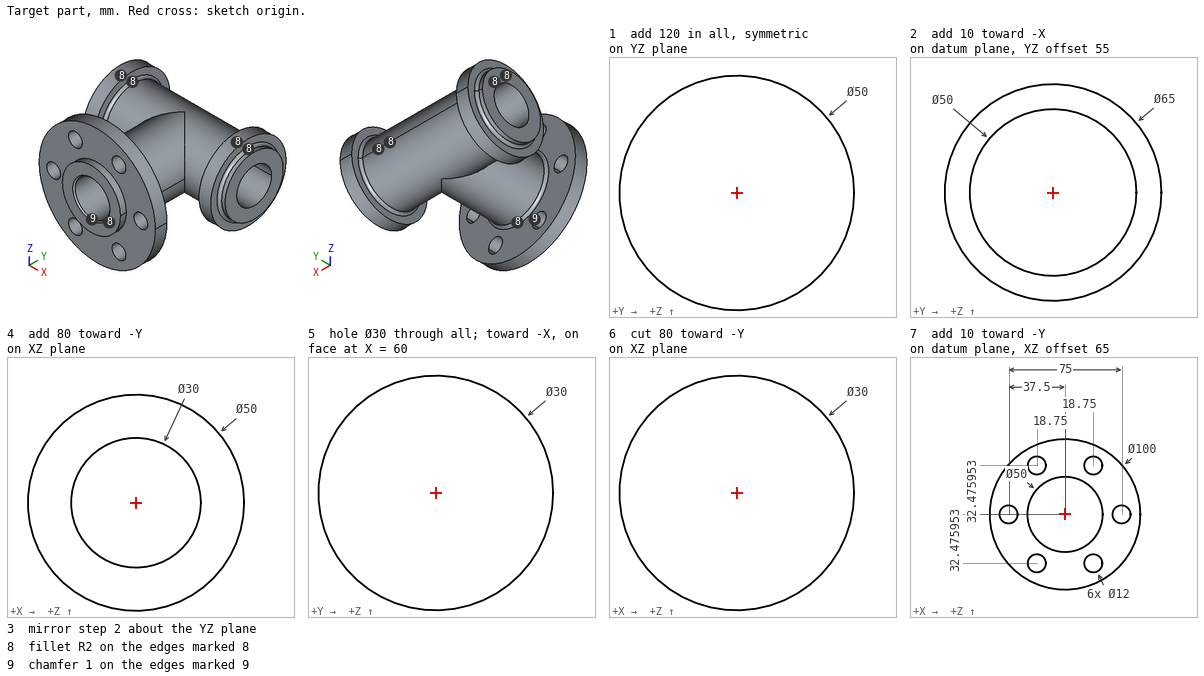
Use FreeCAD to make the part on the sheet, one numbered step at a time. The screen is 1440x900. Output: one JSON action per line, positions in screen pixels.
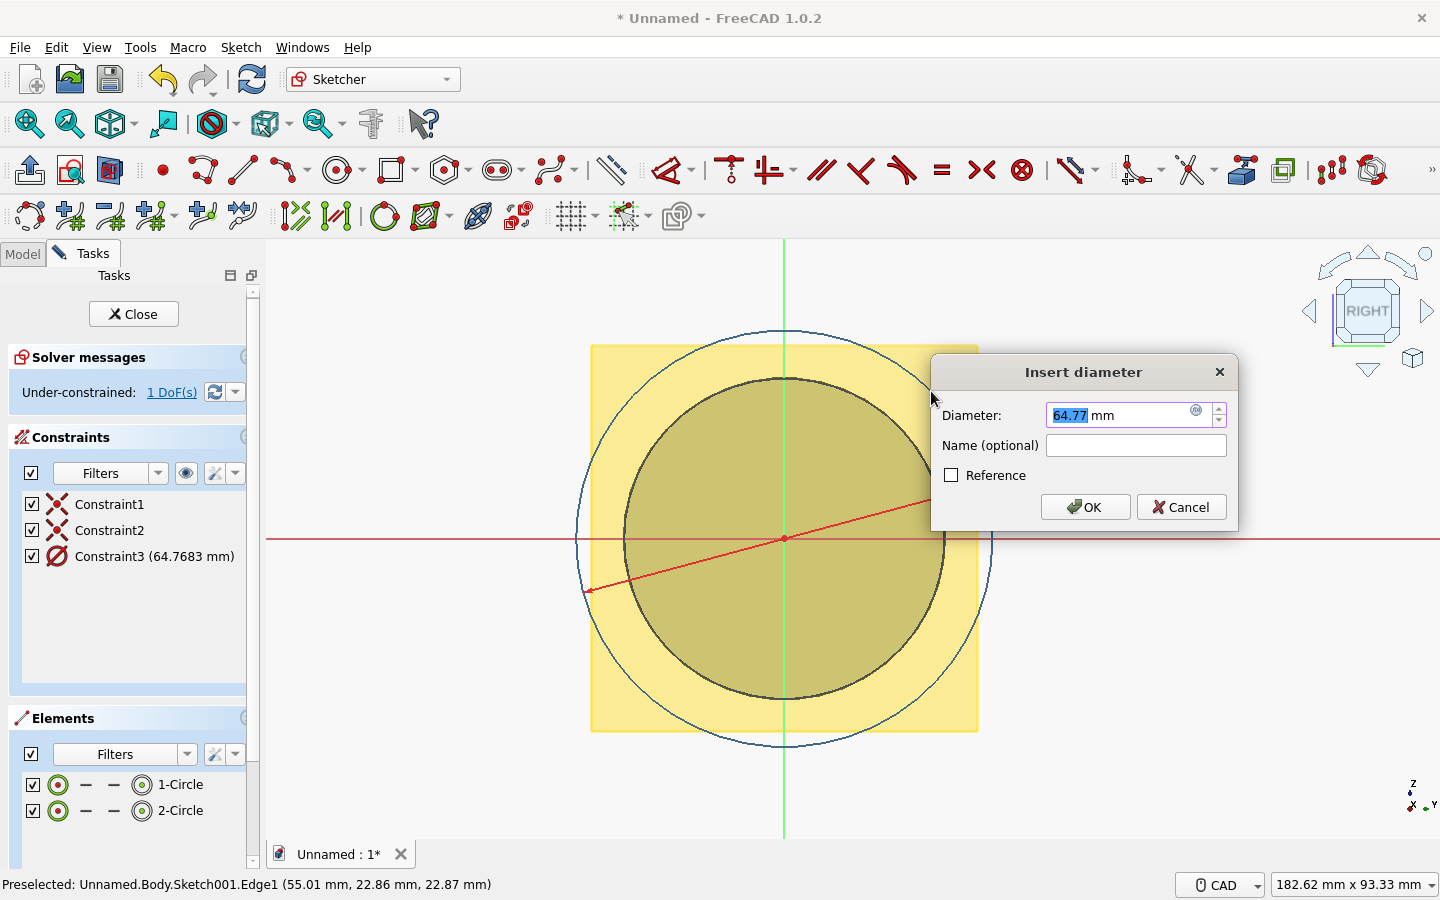
{"action": "type", "text": "65"}
{"action": "key", "text": "Return"}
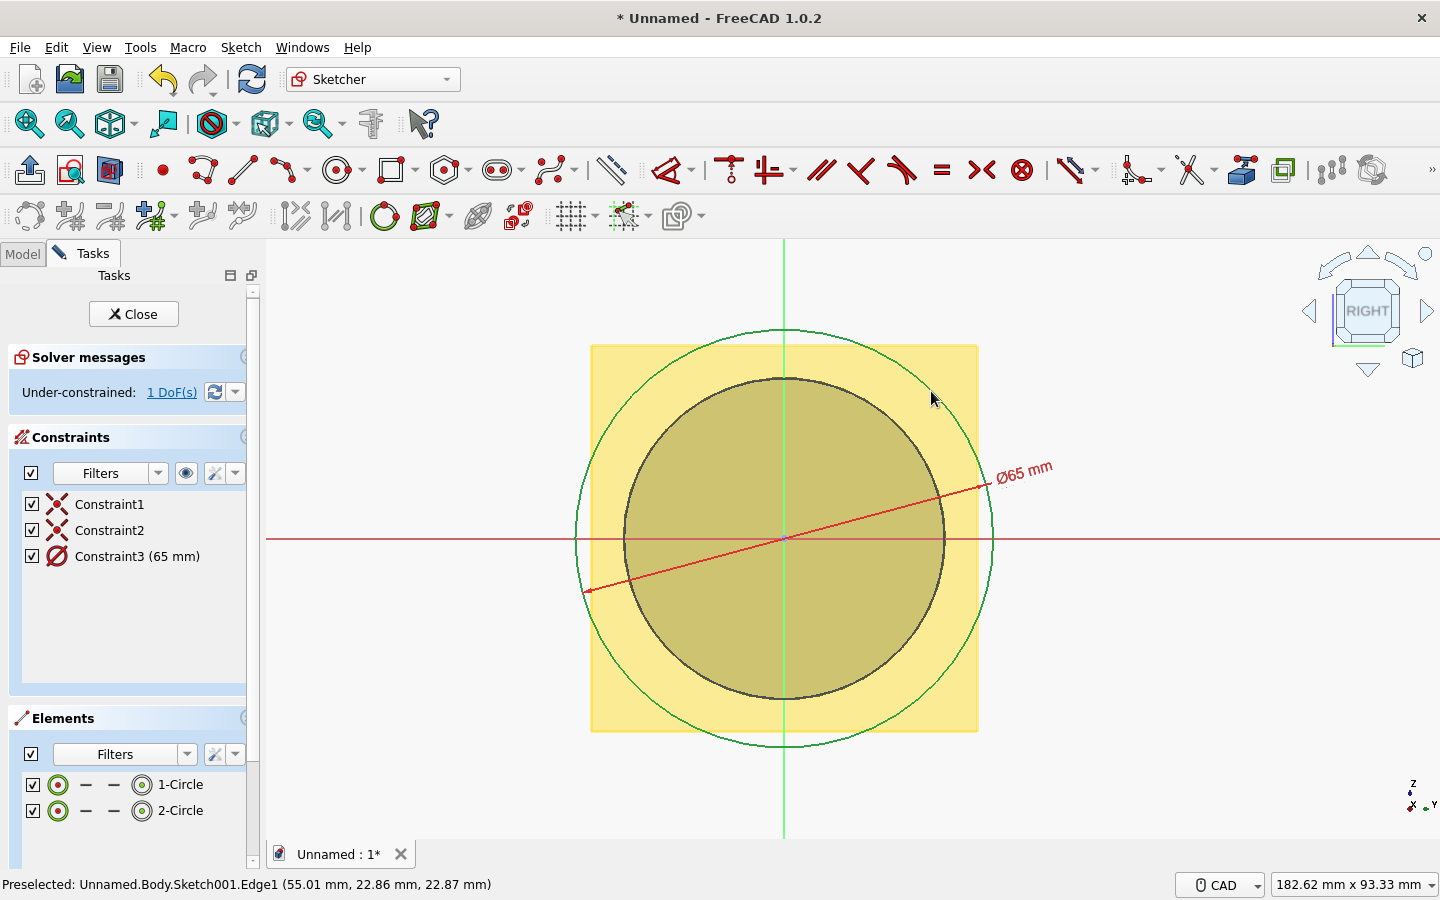
{"action": "left_click", "coordinate": [897, 425]}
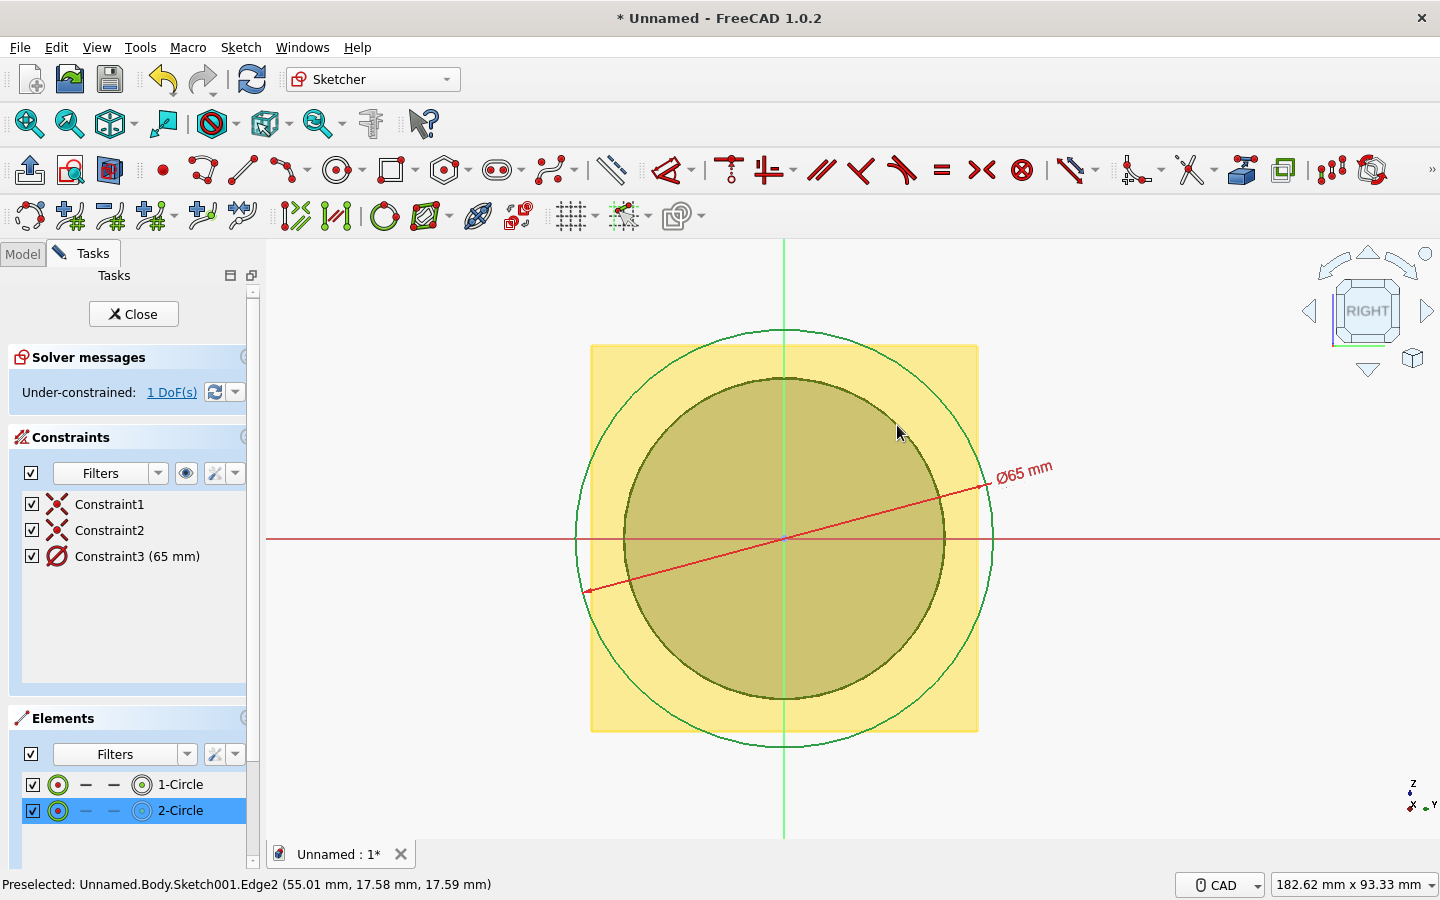
{"action": "key", "text": "k o"}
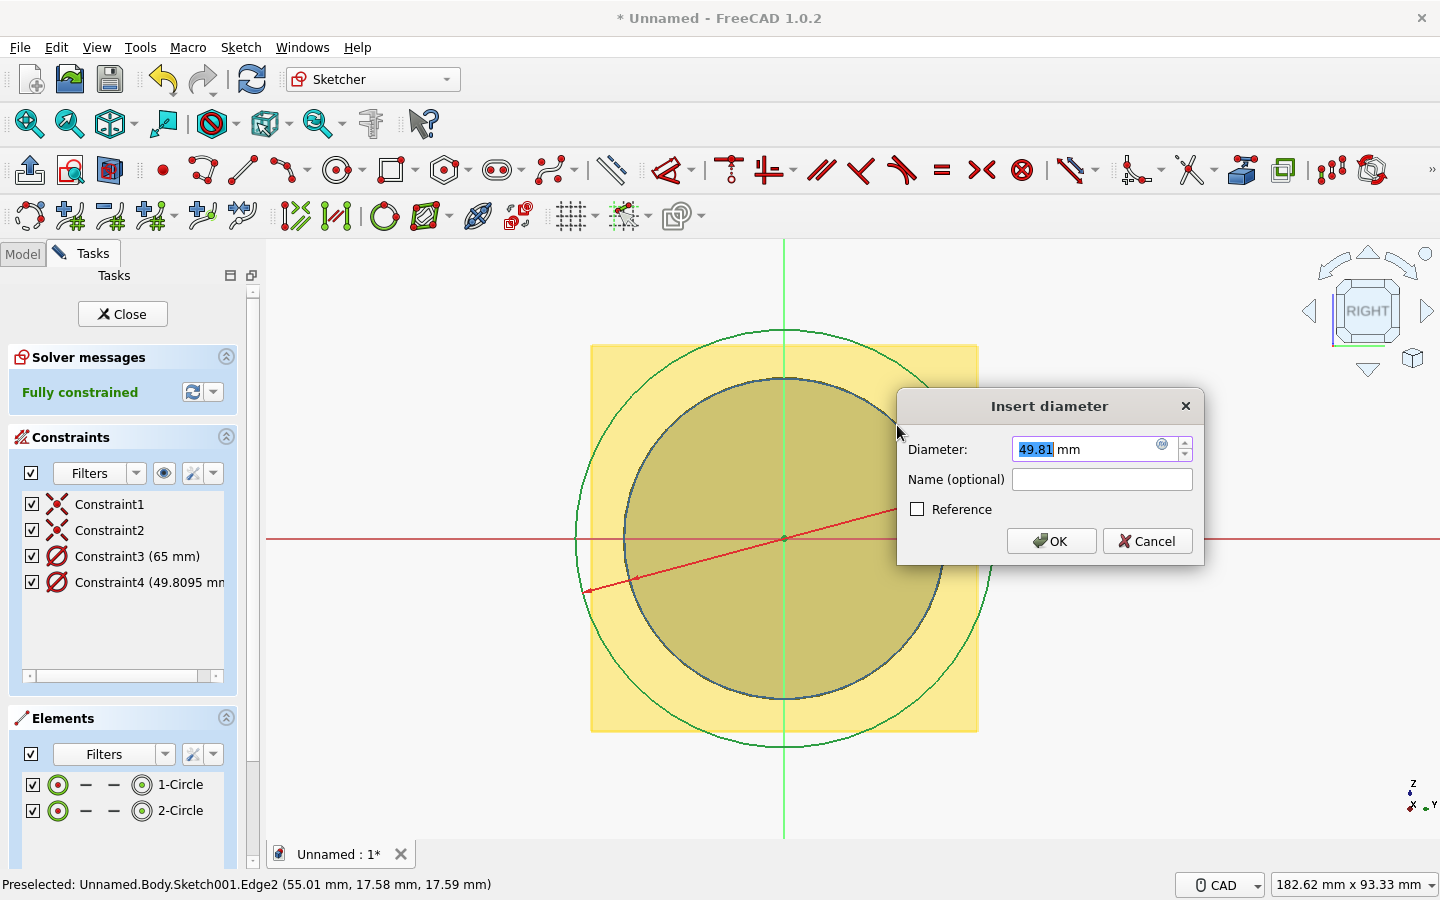
{"action": "type", "text": "50"}
{"action": "key", "text": "Return"}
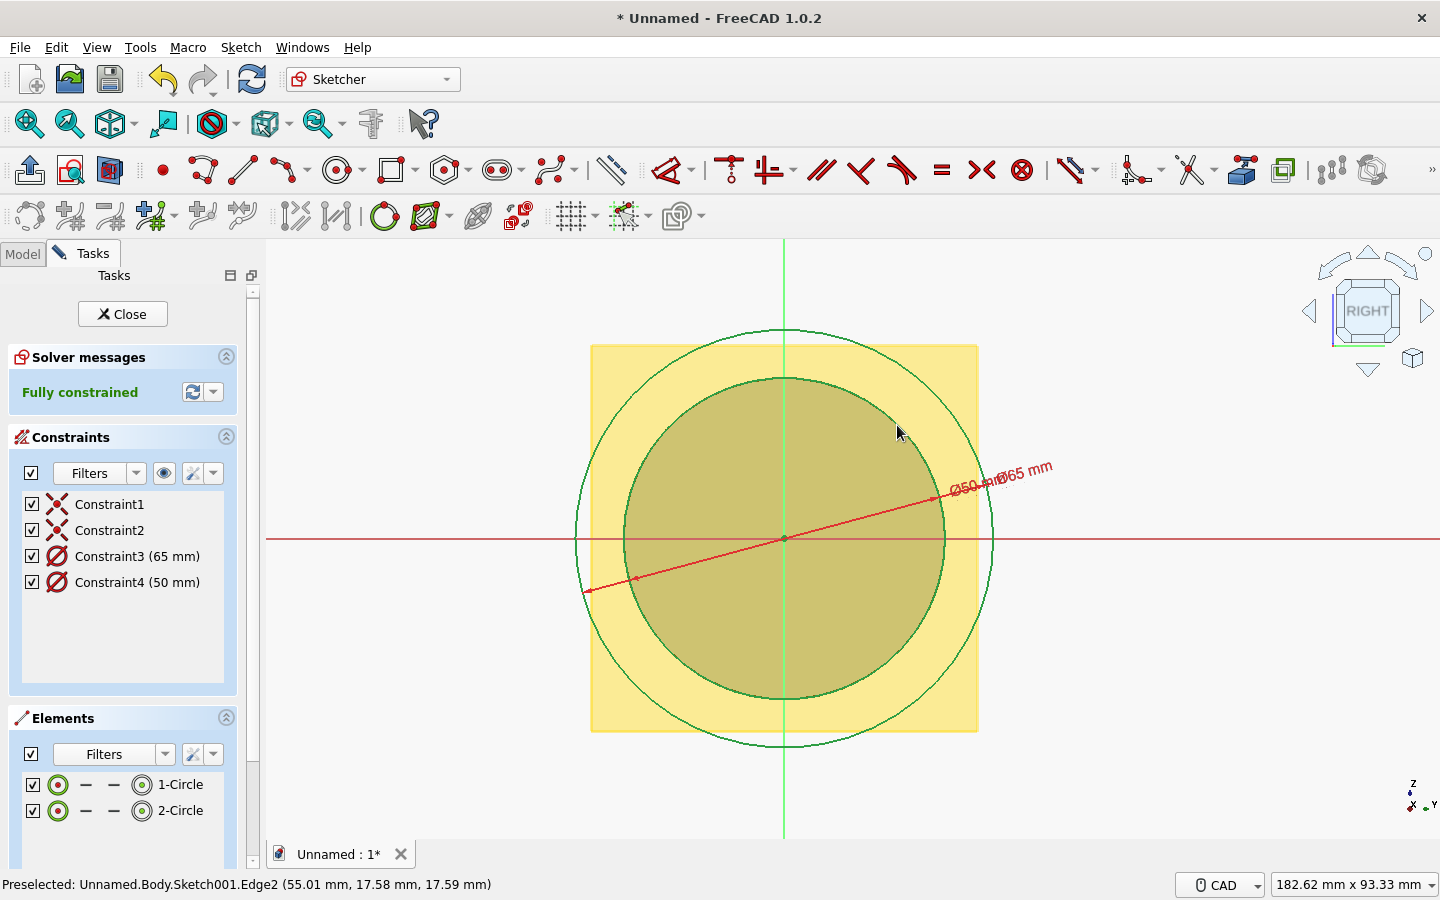
{"action": "left_click", "coordinate": [123, 314]}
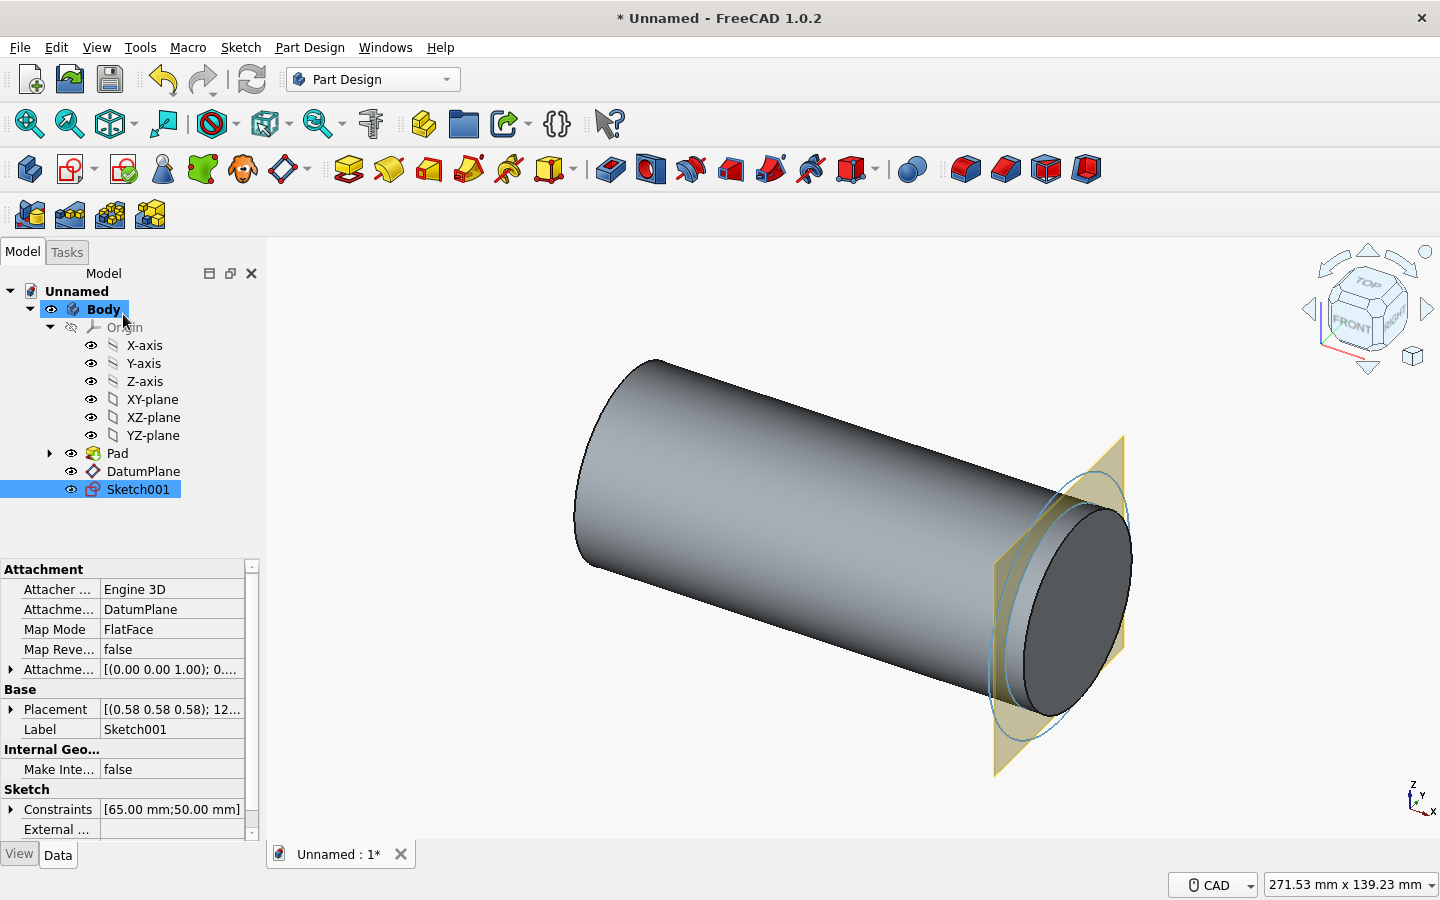
{"action": "left_click", "coordinate": [350, 170]}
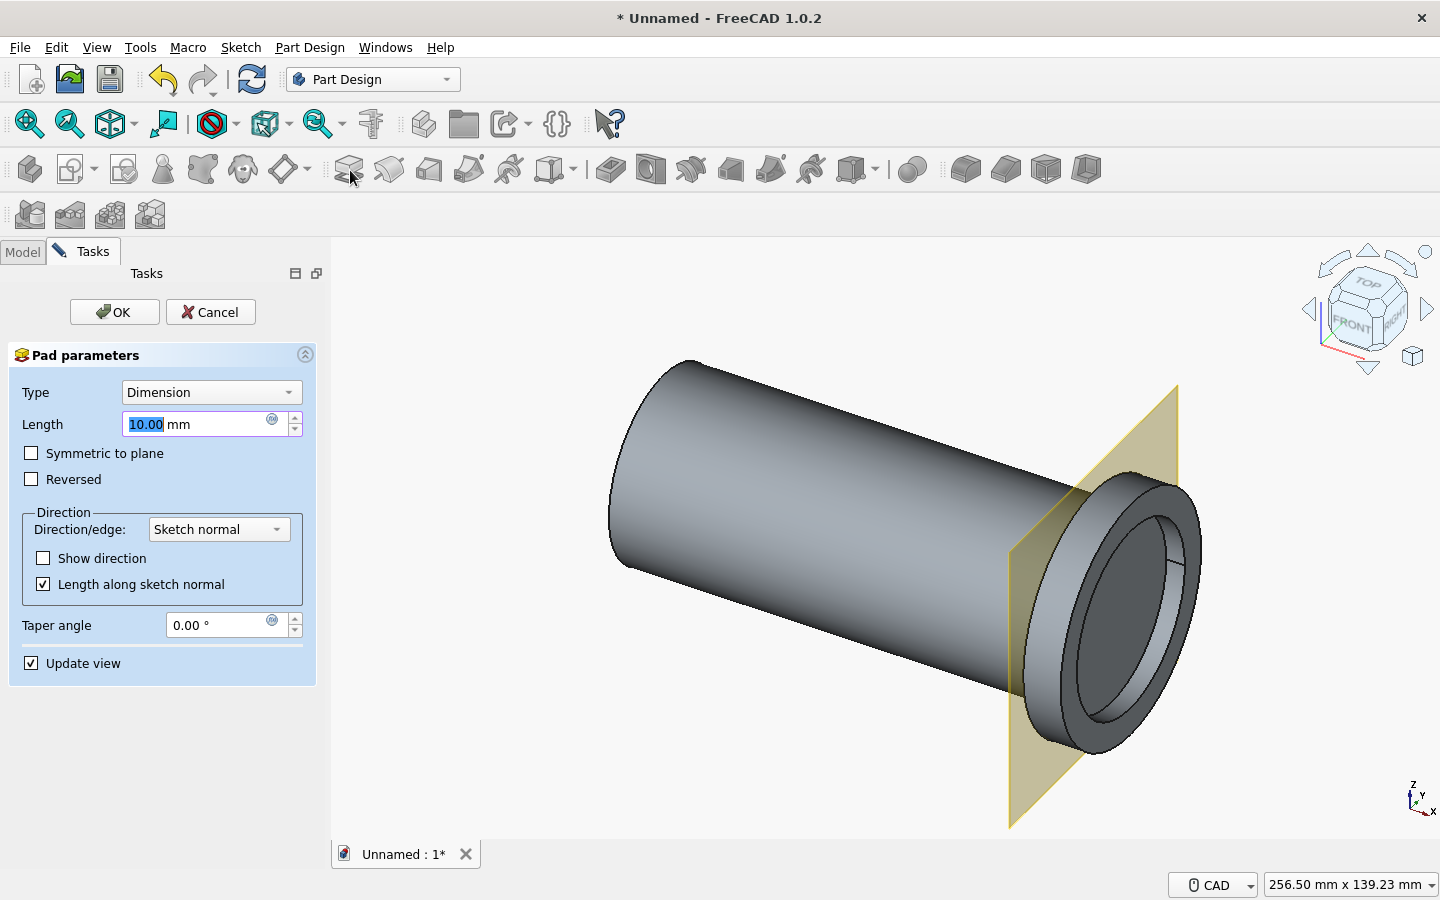
{"action": "type", "text": "10"}
{"action": "key", "text": "Tab"}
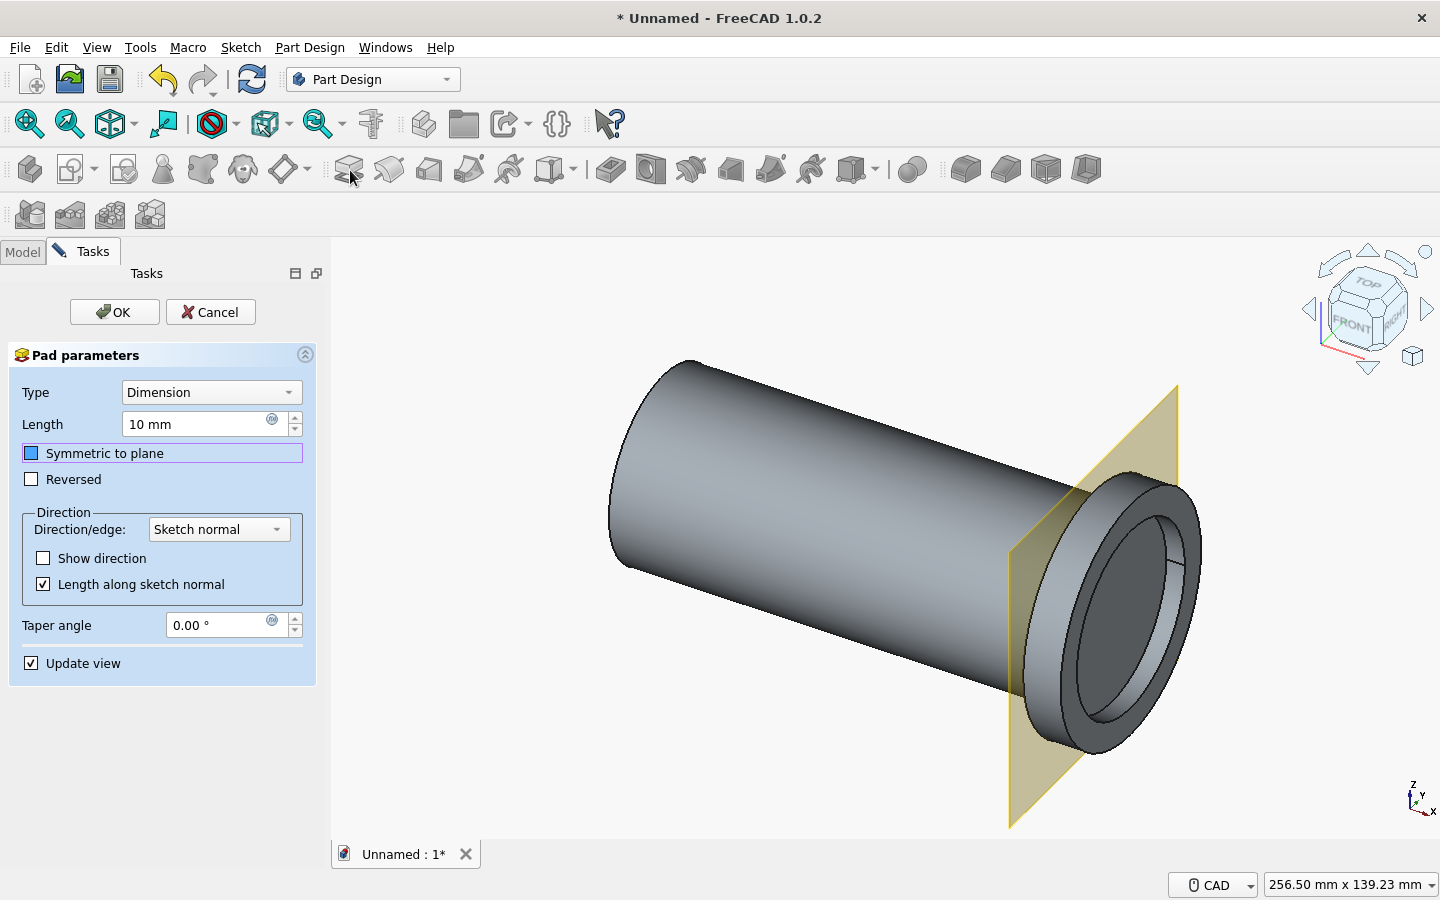
{"action": "left_click", "coordinate": [30, 479]}